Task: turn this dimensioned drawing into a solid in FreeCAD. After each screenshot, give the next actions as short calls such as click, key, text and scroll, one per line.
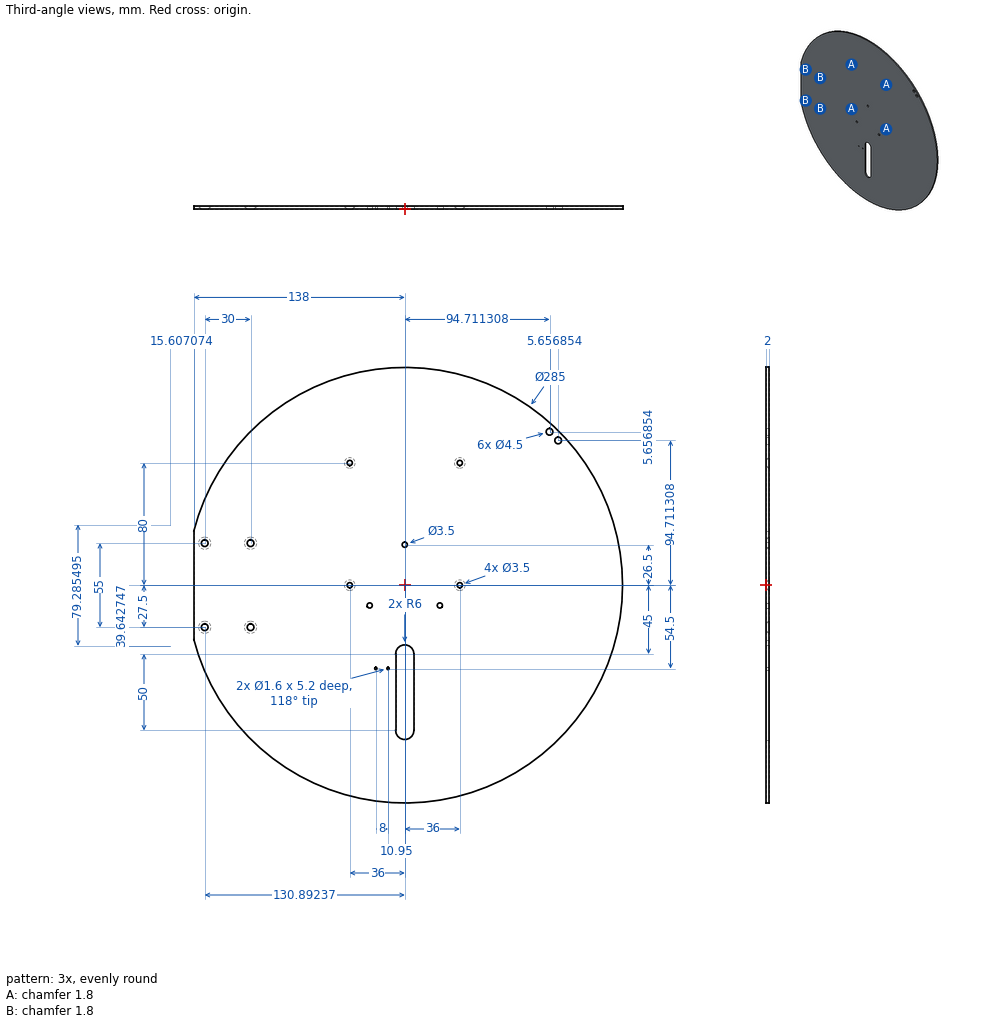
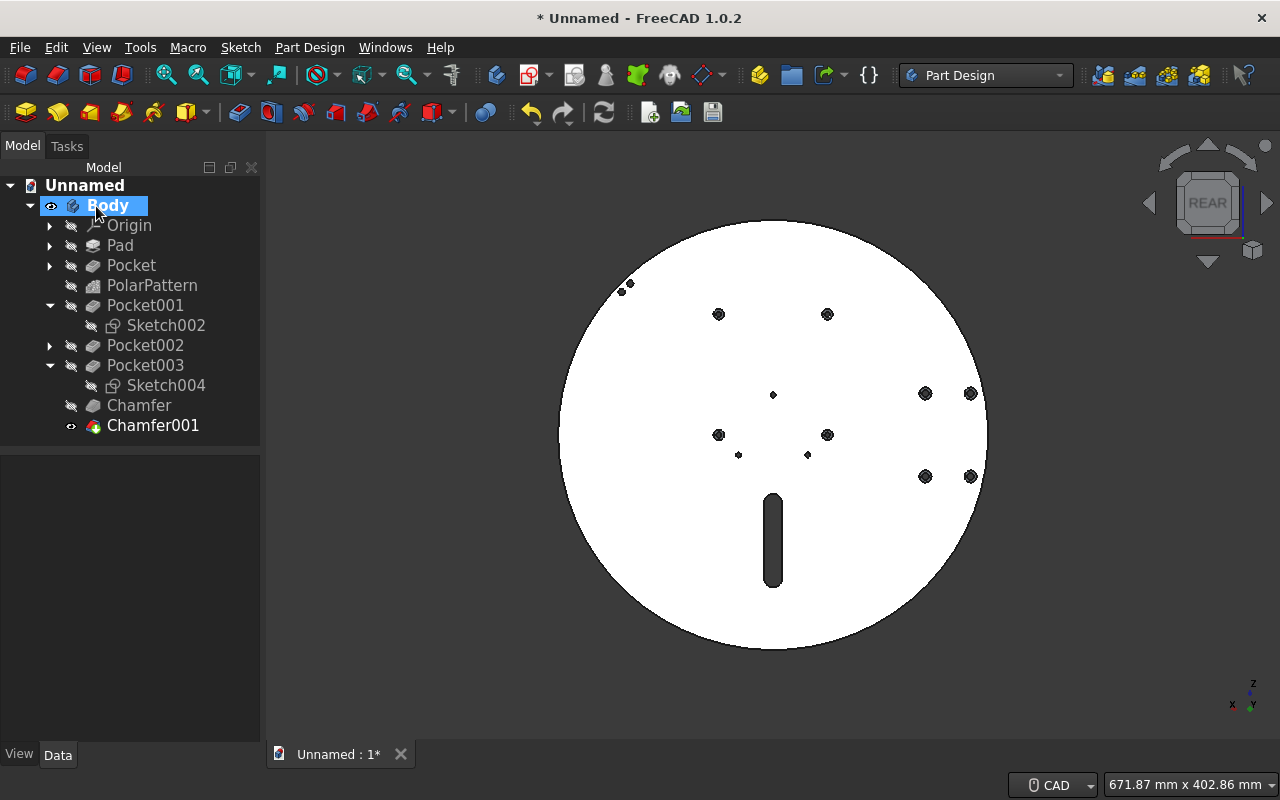
key(0)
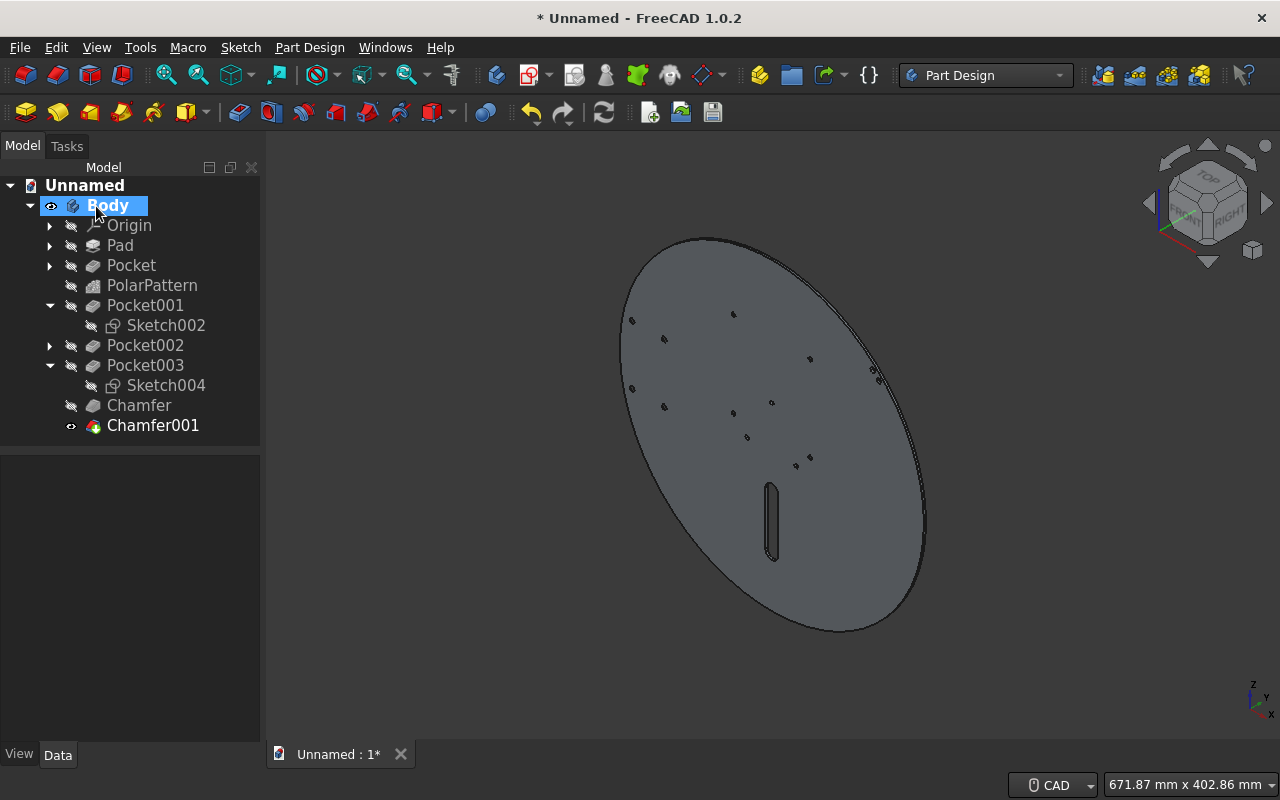
click(859, 535)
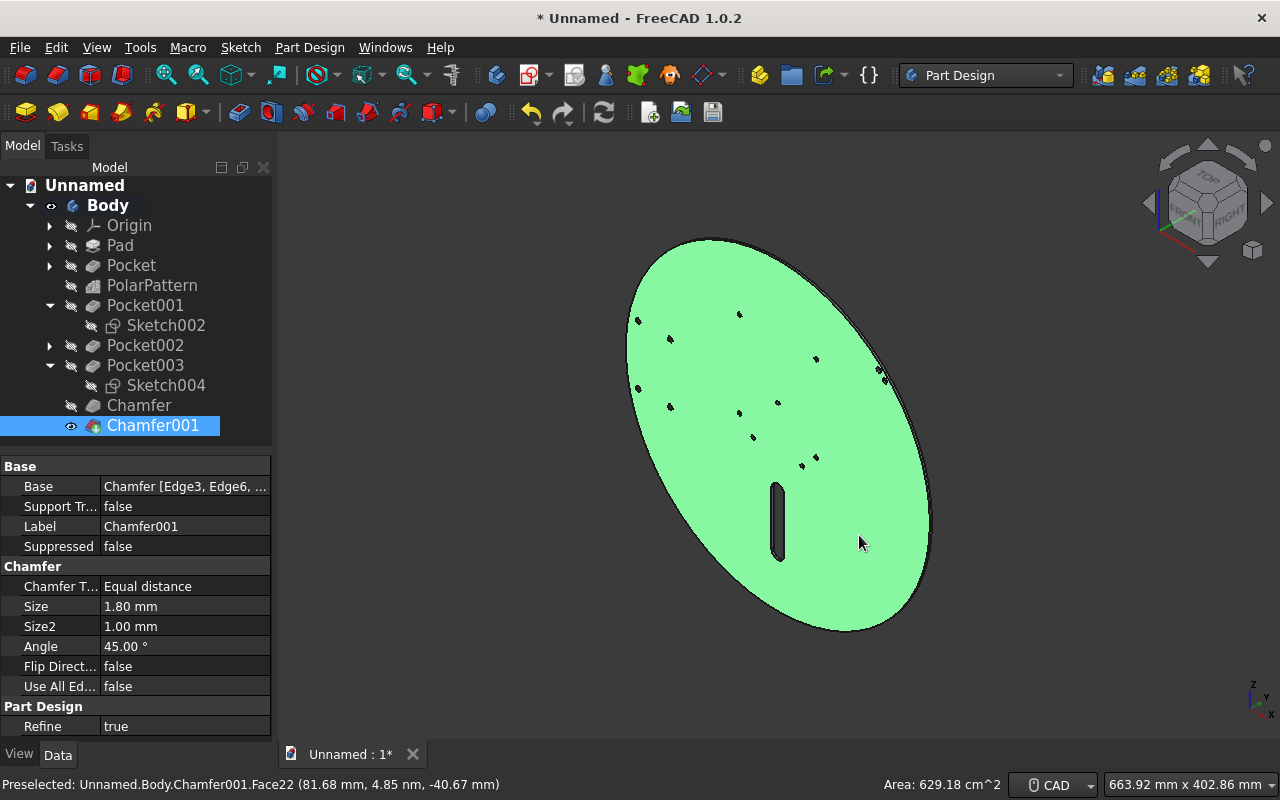
click(530, 76)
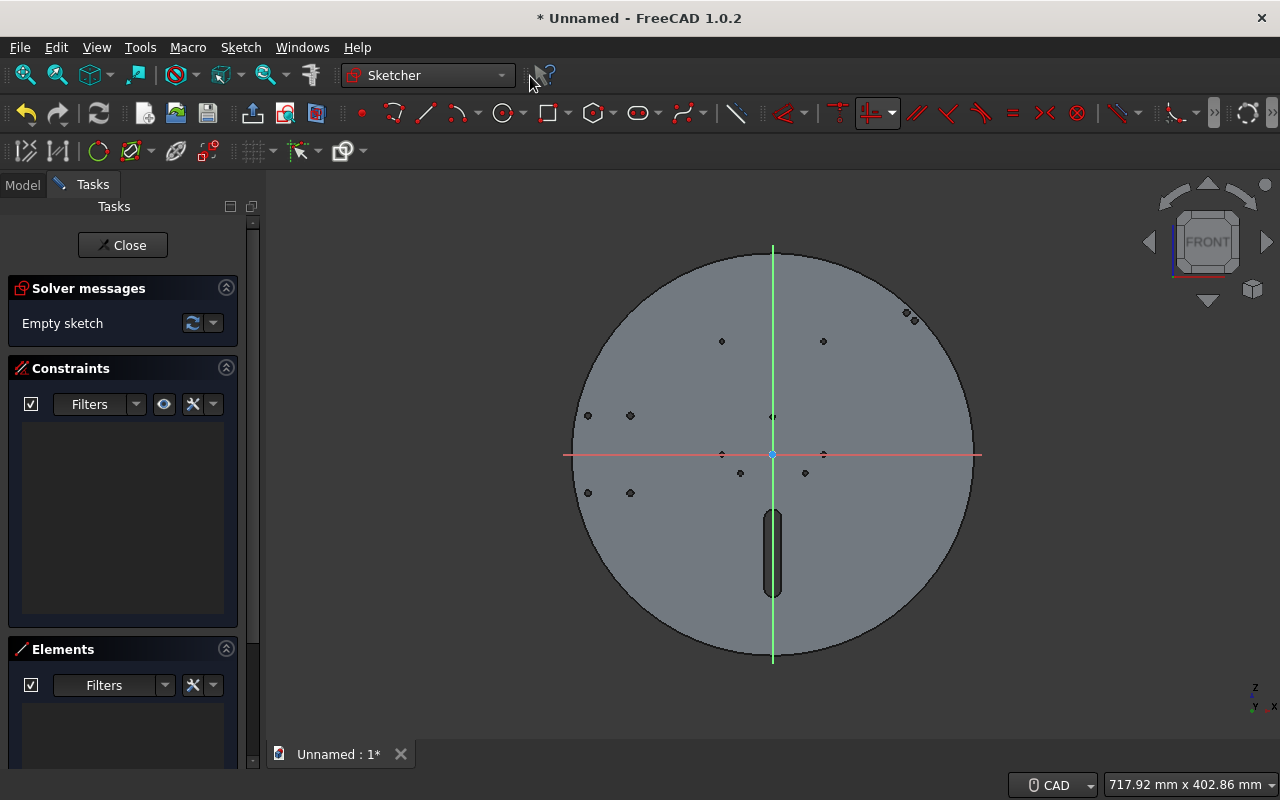
scroll(754, 536, up, 15)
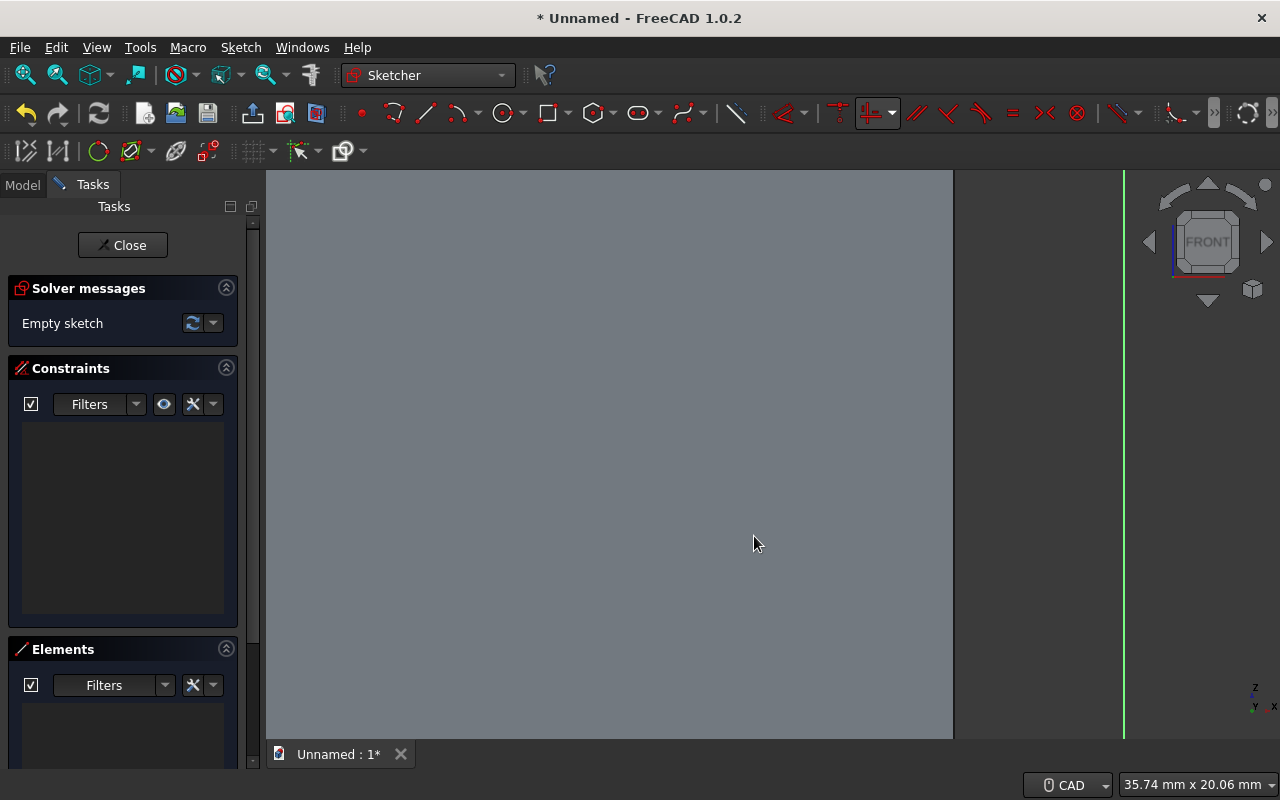
scroll(696, 415, up, 4)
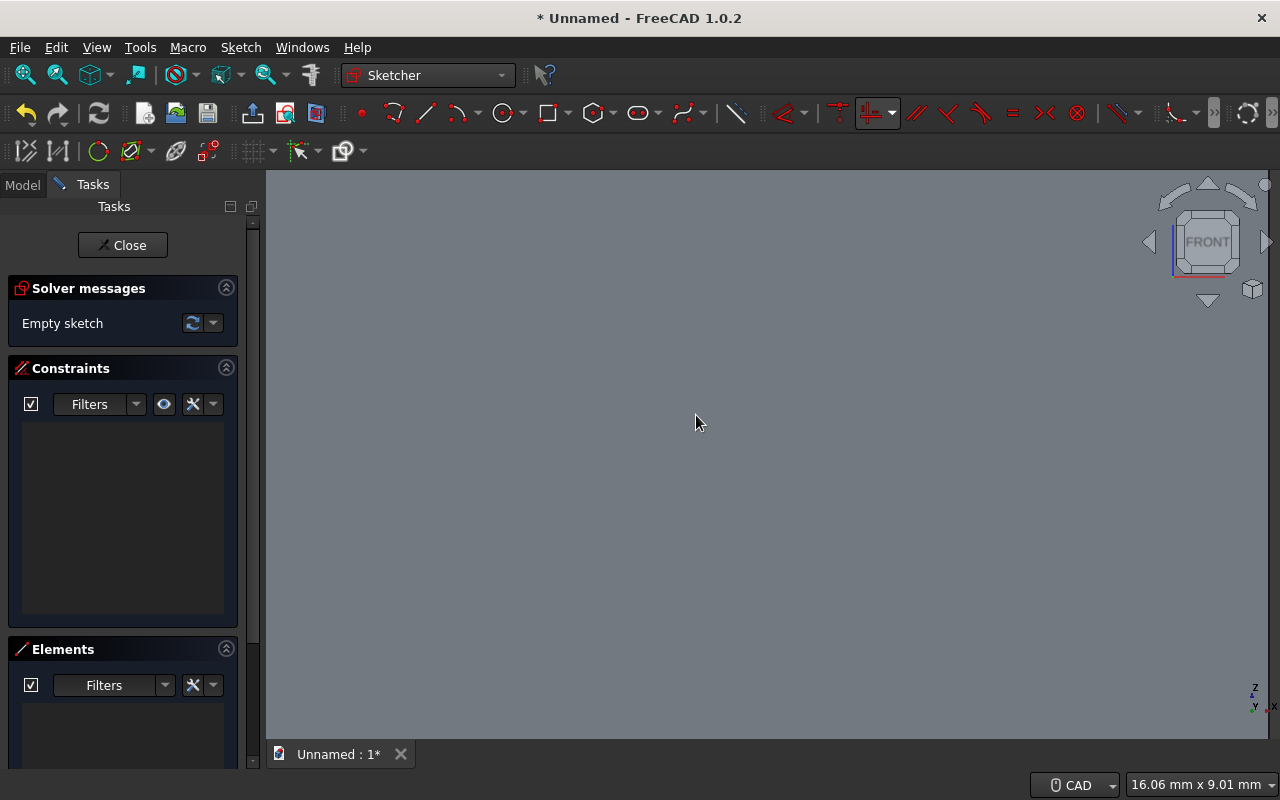
click(504, 114)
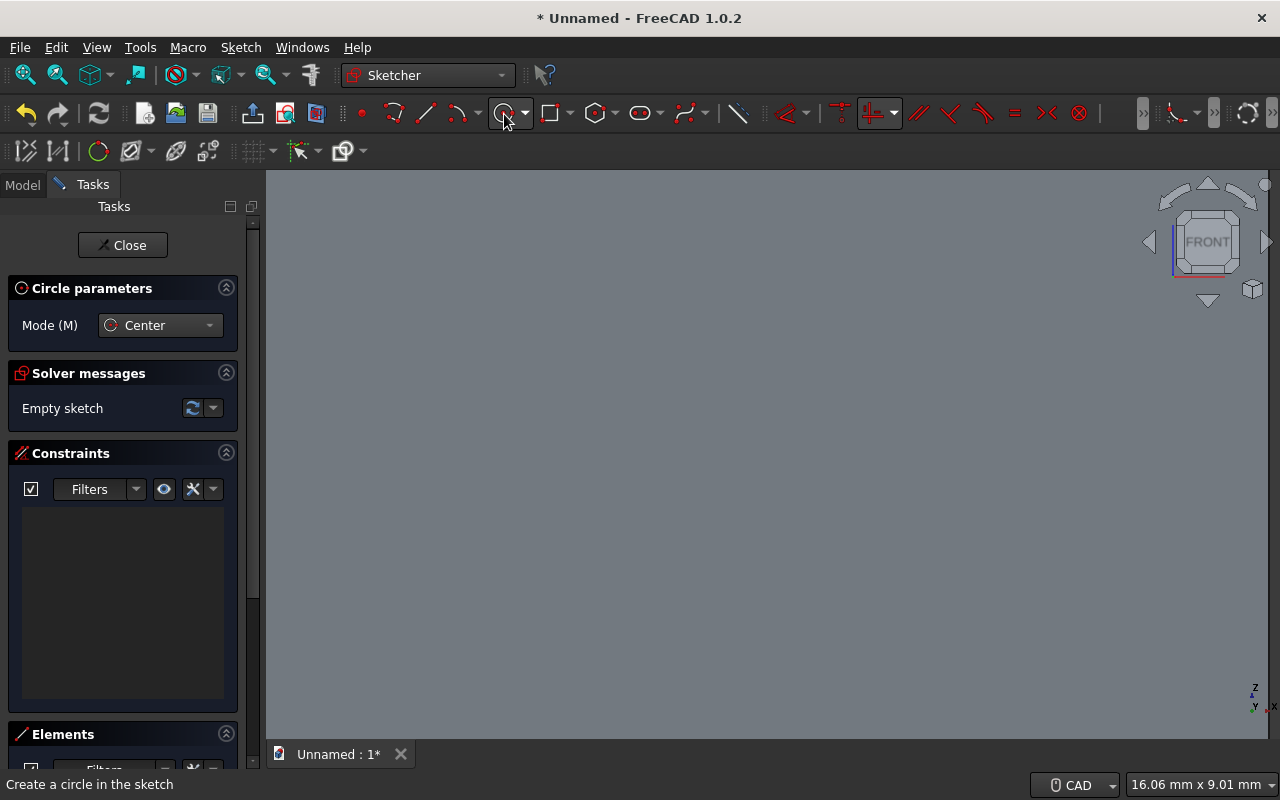
click(956, 454)
click(992, 418)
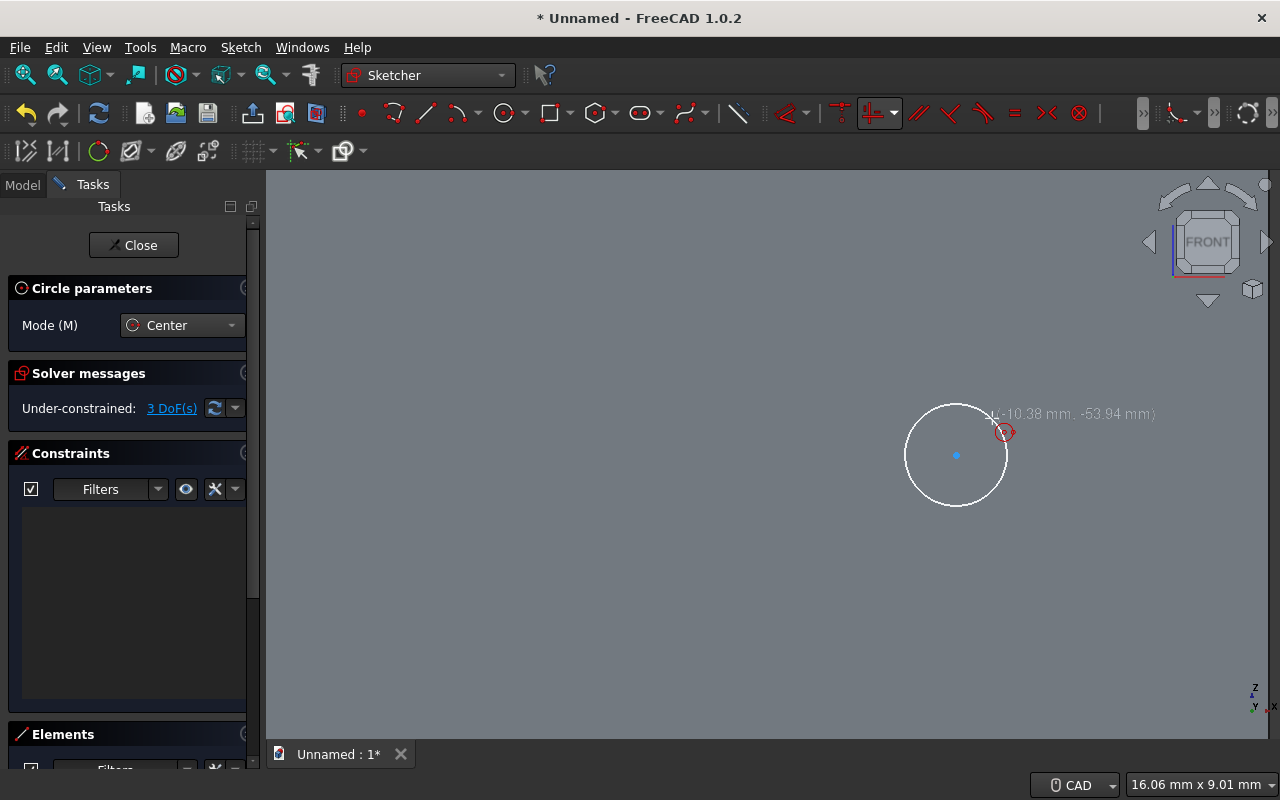
click(451, 454)
click(487, 418)
key(Escape)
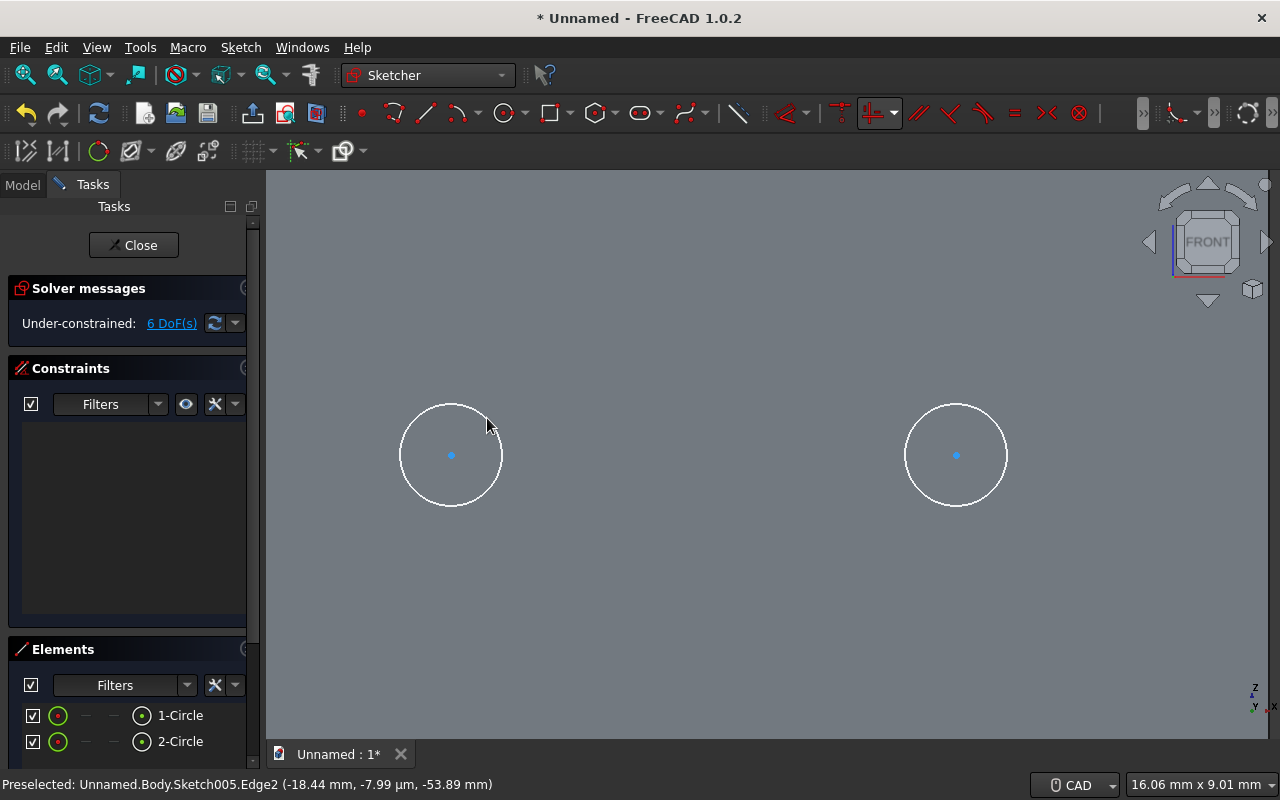
click(992, 419)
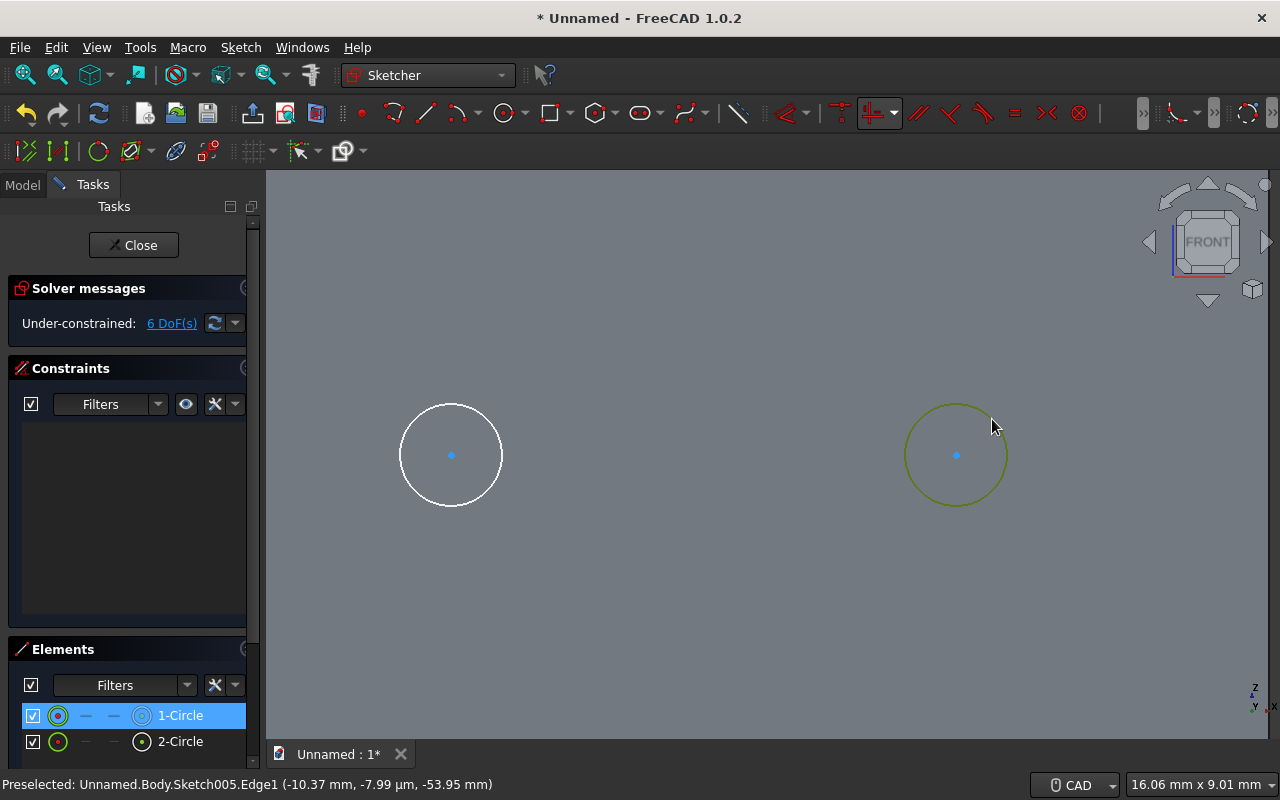
click(487, 419)